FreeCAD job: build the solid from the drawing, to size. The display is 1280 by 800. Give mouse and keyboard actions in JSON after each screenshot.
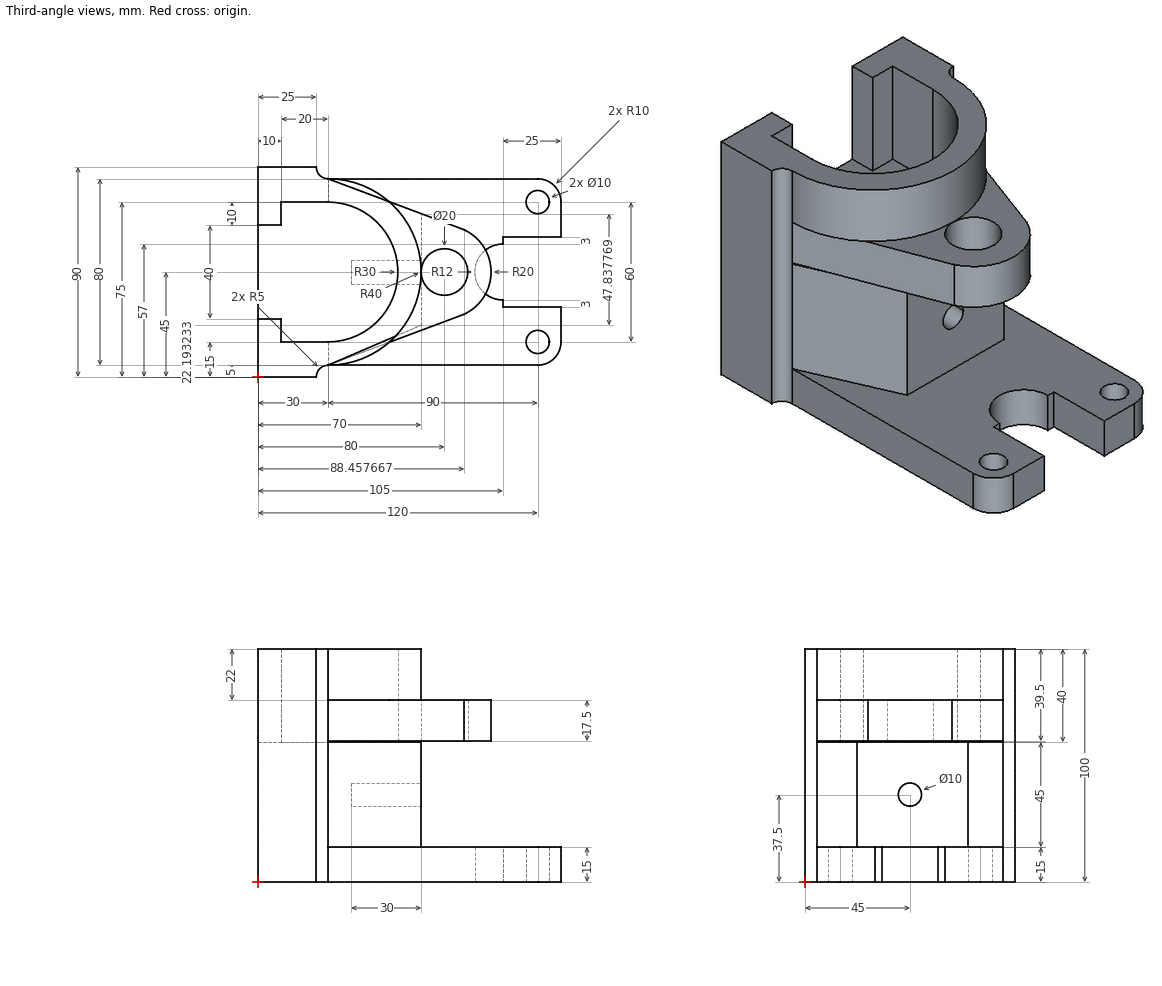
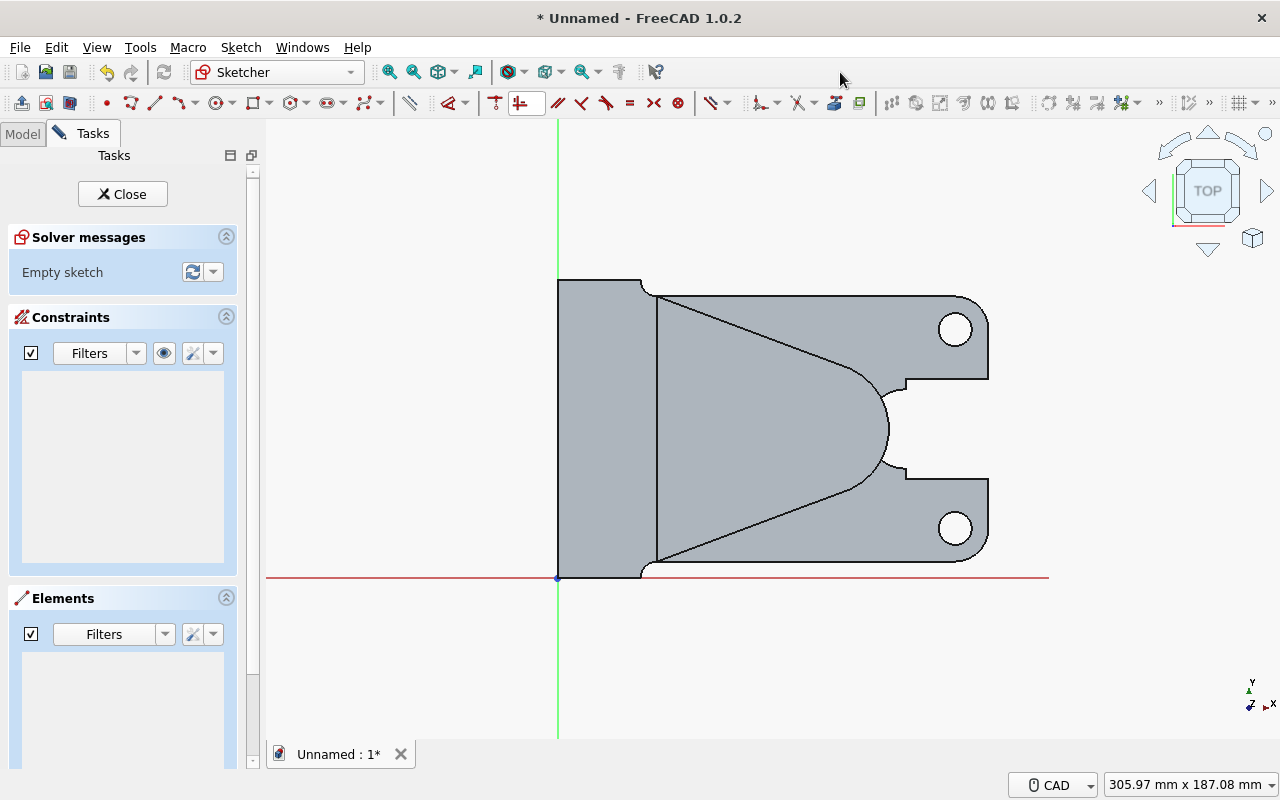
{"action": "scroll", "coordinate": [846, 429], "scroll_direction": "up", "scroll_amount": 9}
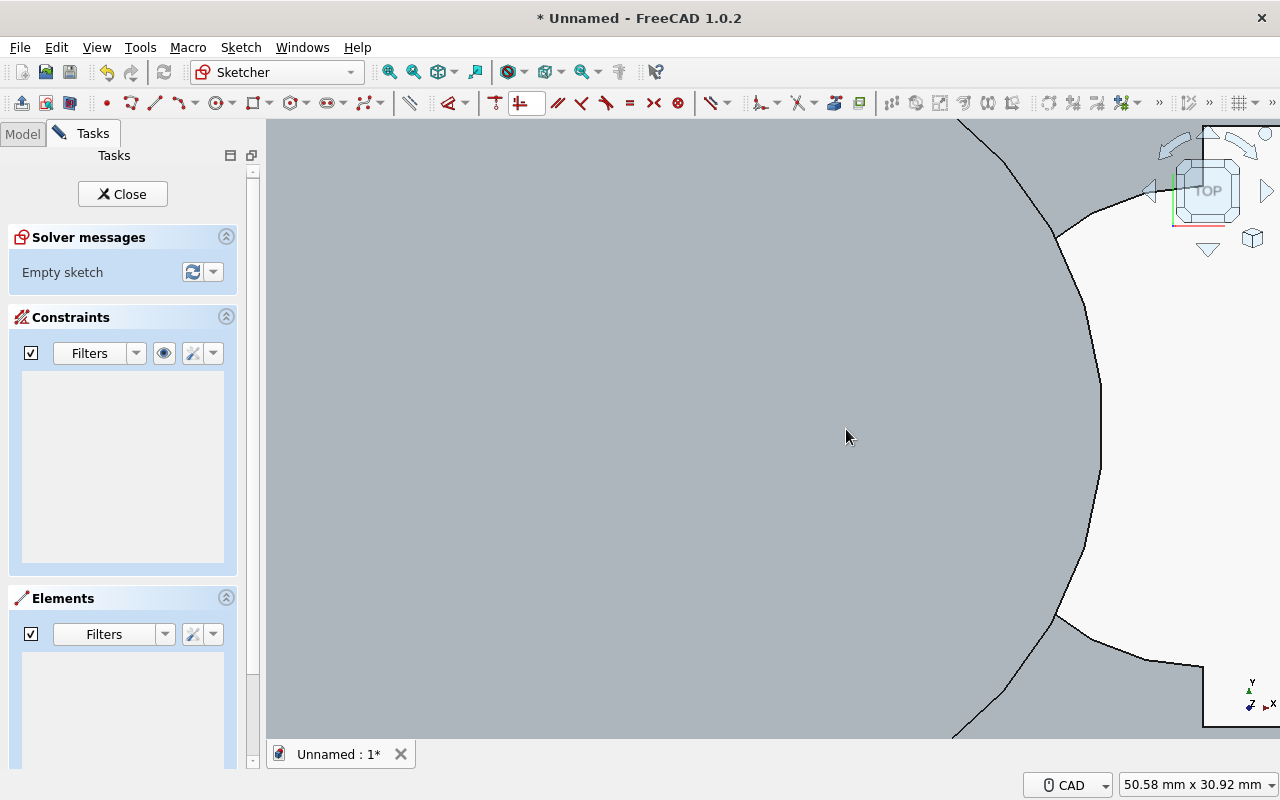
{"action": "left_click", "coordinate": [216, 104]}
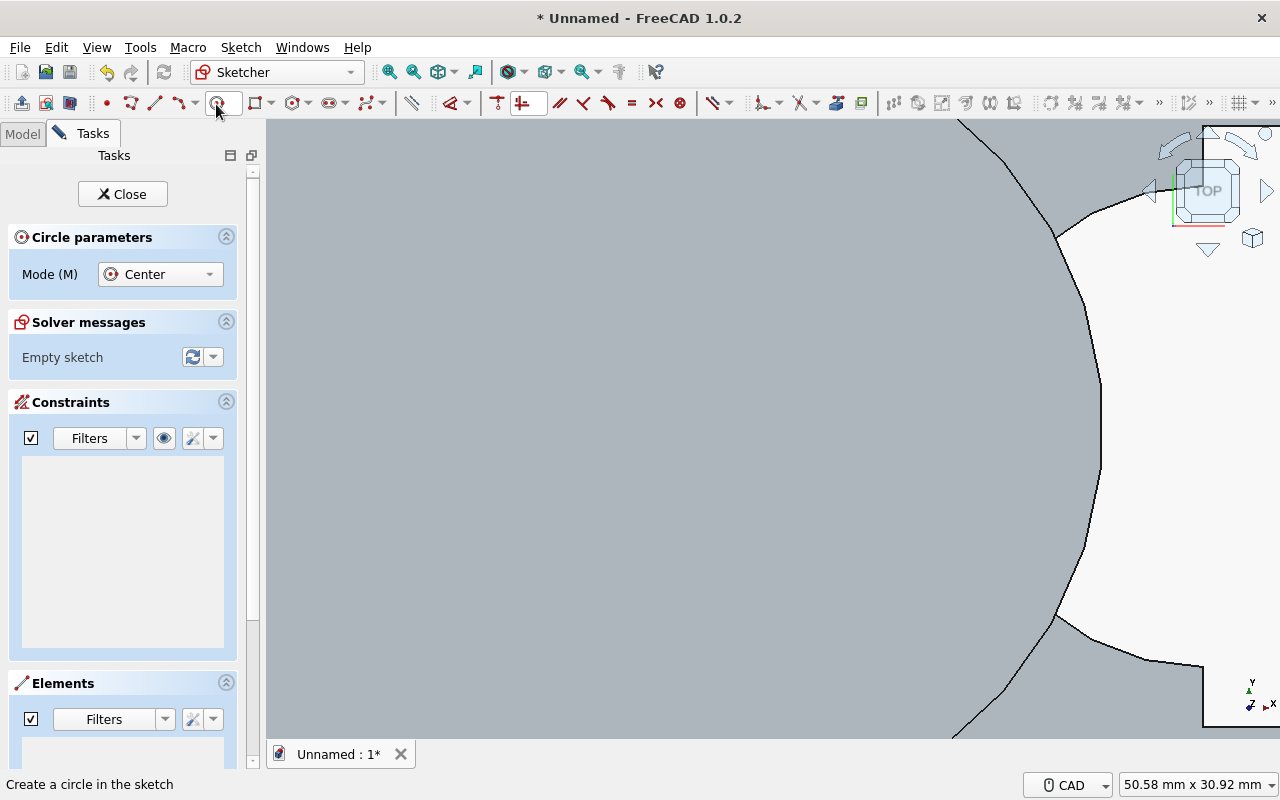
{"action": "left_click", "coordinate": [702, 426]}
{"action": "left_click", "coordinate": [844, 285]}
{"action": "key", "text": "Escape"}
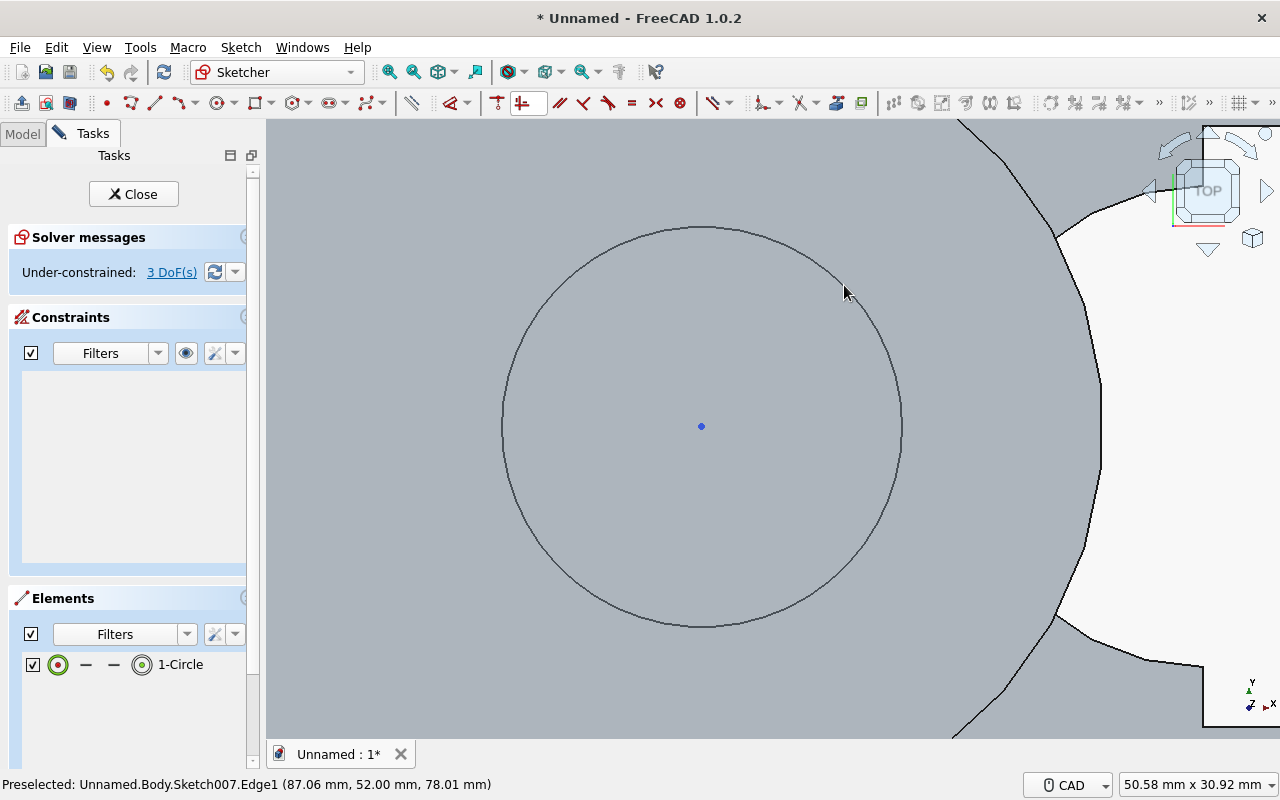
{"action": "left_click", "coordinate": [450, 104]}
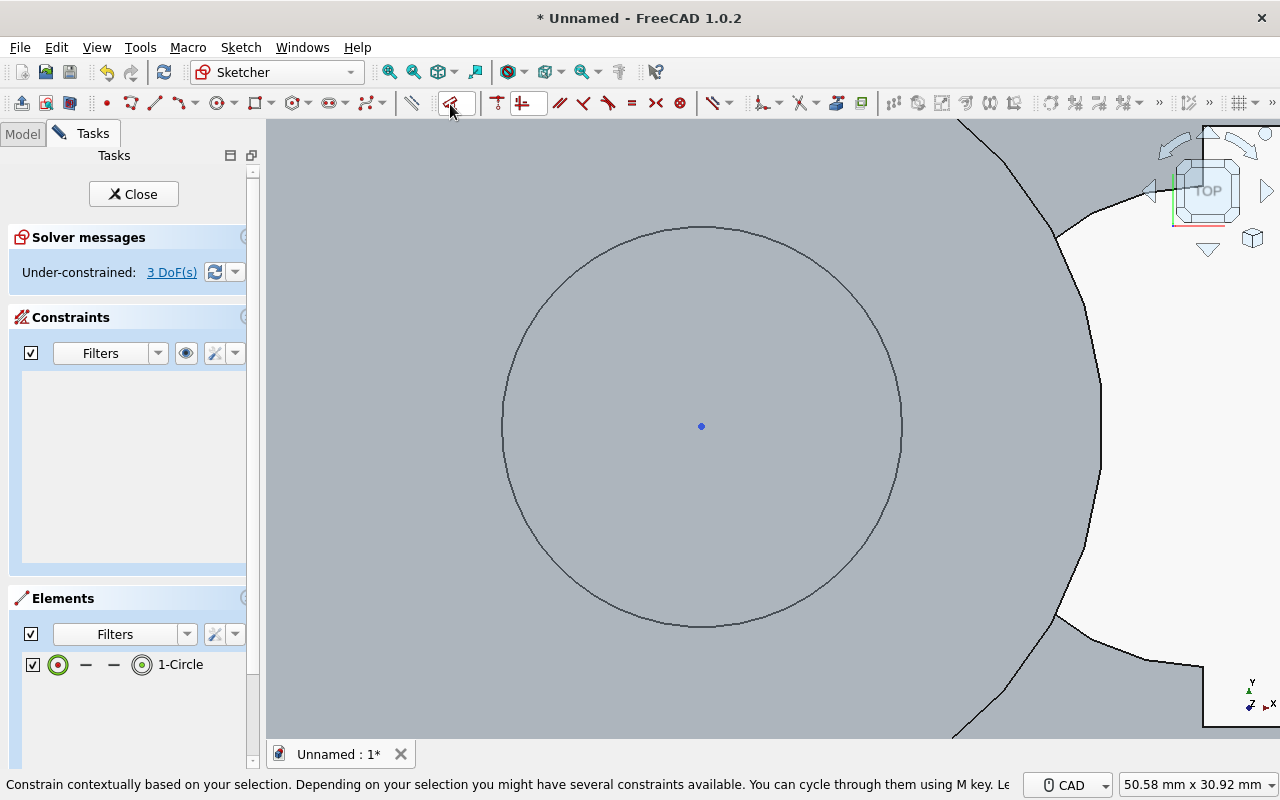
{"action": "left_click", "coordinate": [843, 285]}
{"action": "left_click", "coordinate": [866, 262]}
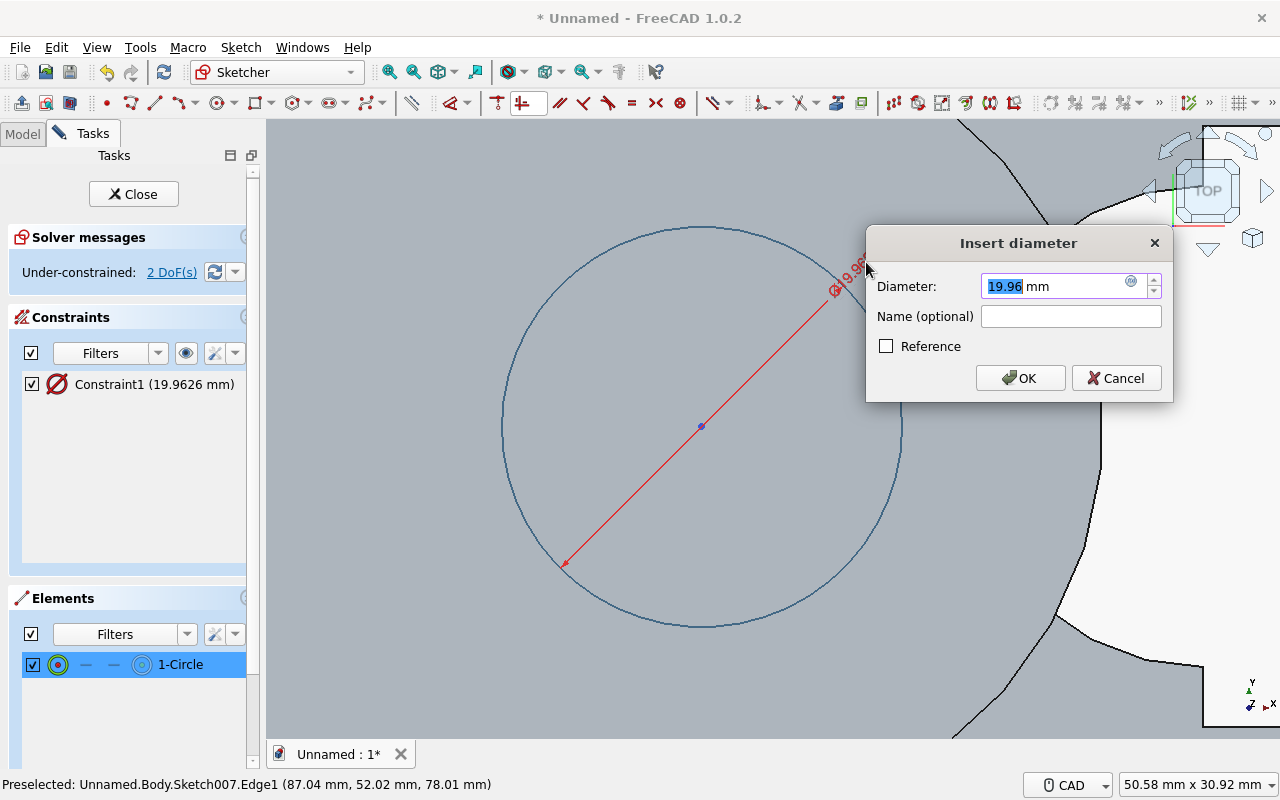
{"action": "type", "text": "20"}
{"action": "key", "text": "Return"}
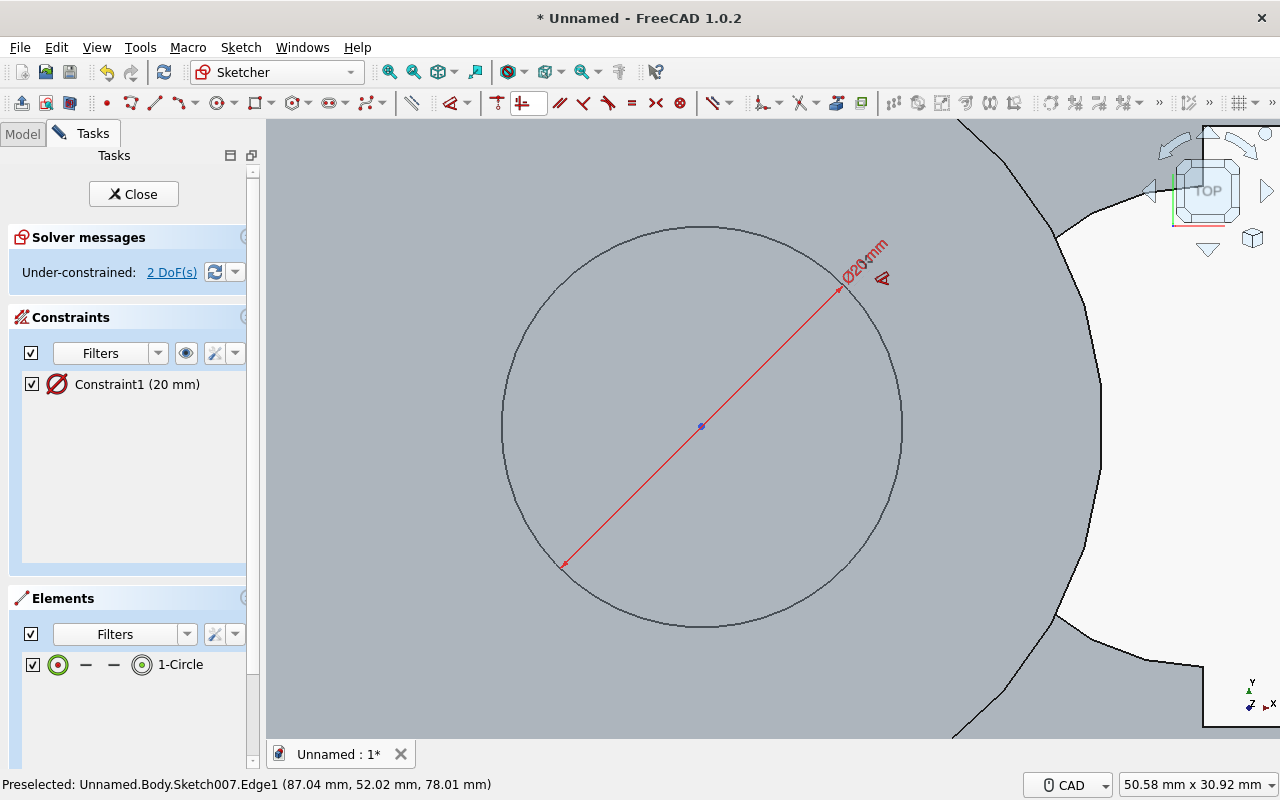
{"action": "left_click", "coordinate": [702, 427]}
{"action": "left_click", "coordinate": [404, 393]}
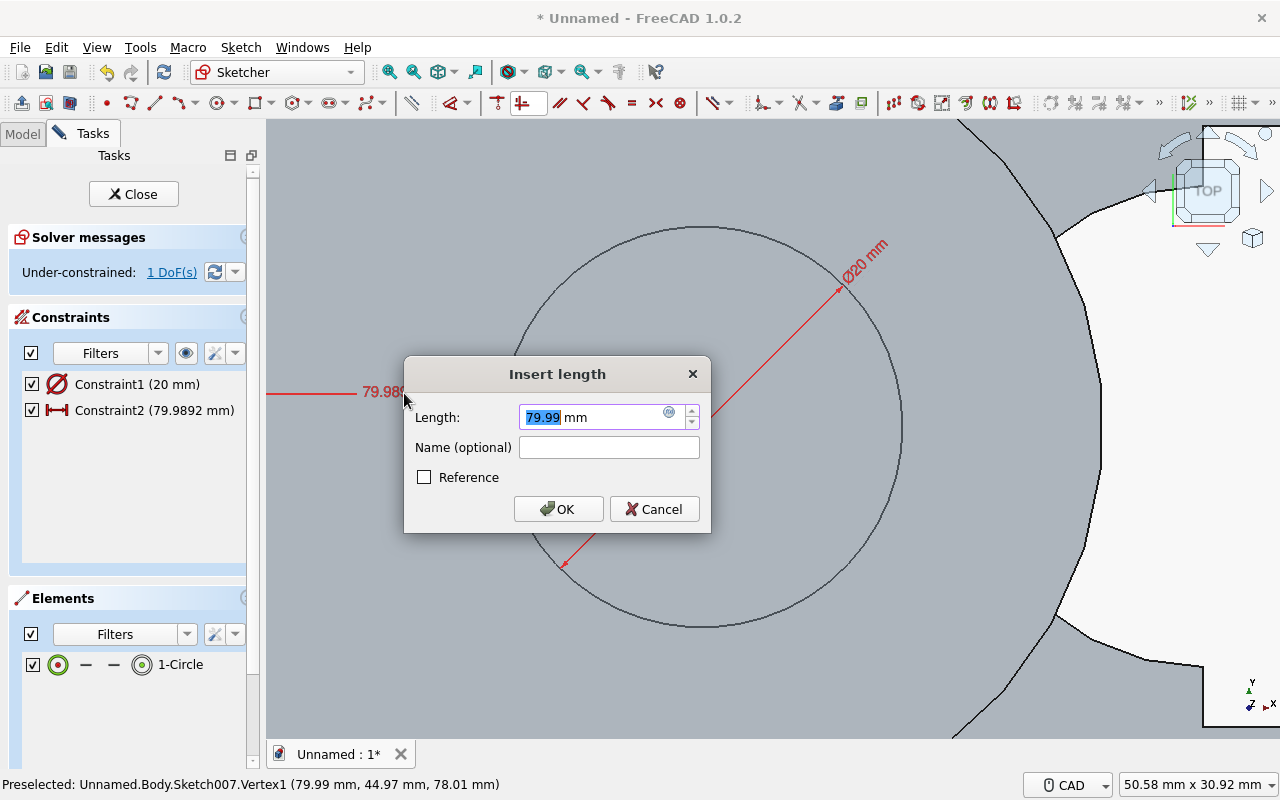
{"action": "type", "text": "80"}
{"action": "key", "text": "Return"}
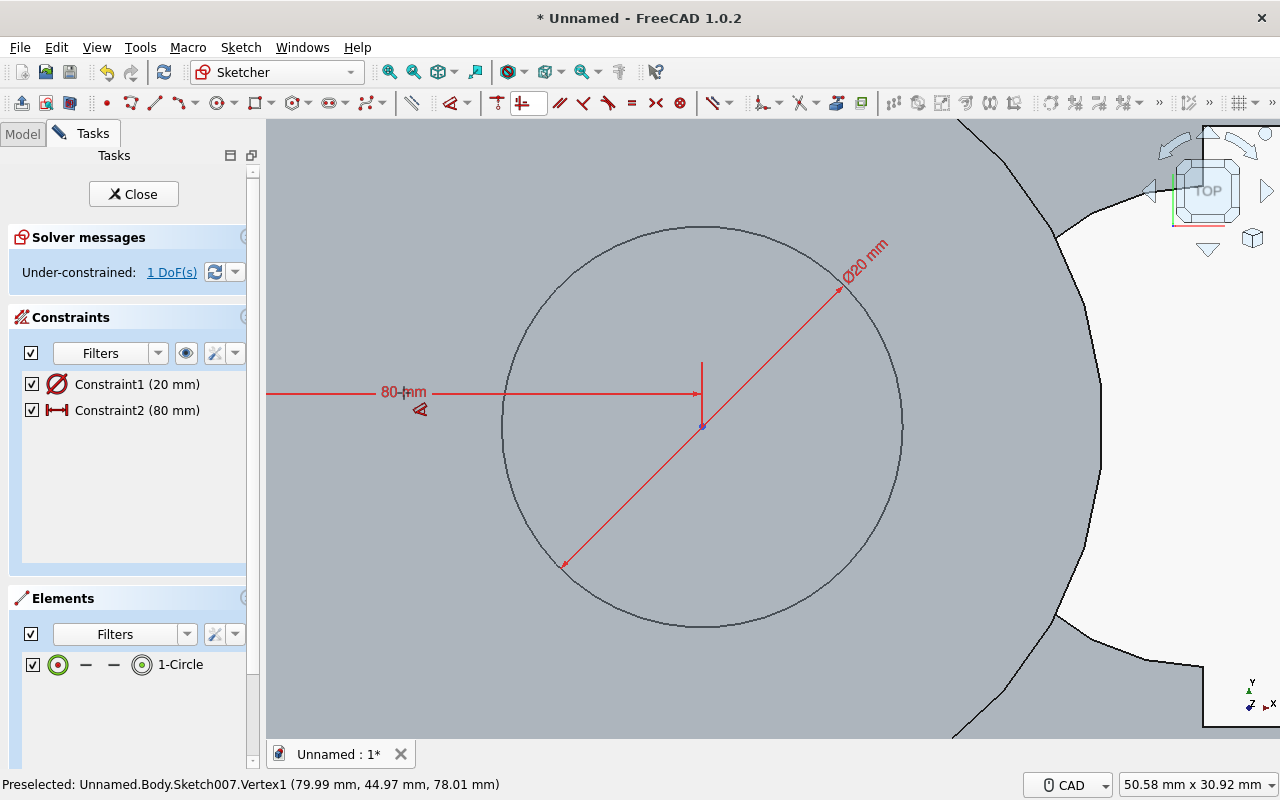
{"action": "left_click", "coordinate": [702, 427]}
{"action": "left_click", "coordinate": [736, 569]}